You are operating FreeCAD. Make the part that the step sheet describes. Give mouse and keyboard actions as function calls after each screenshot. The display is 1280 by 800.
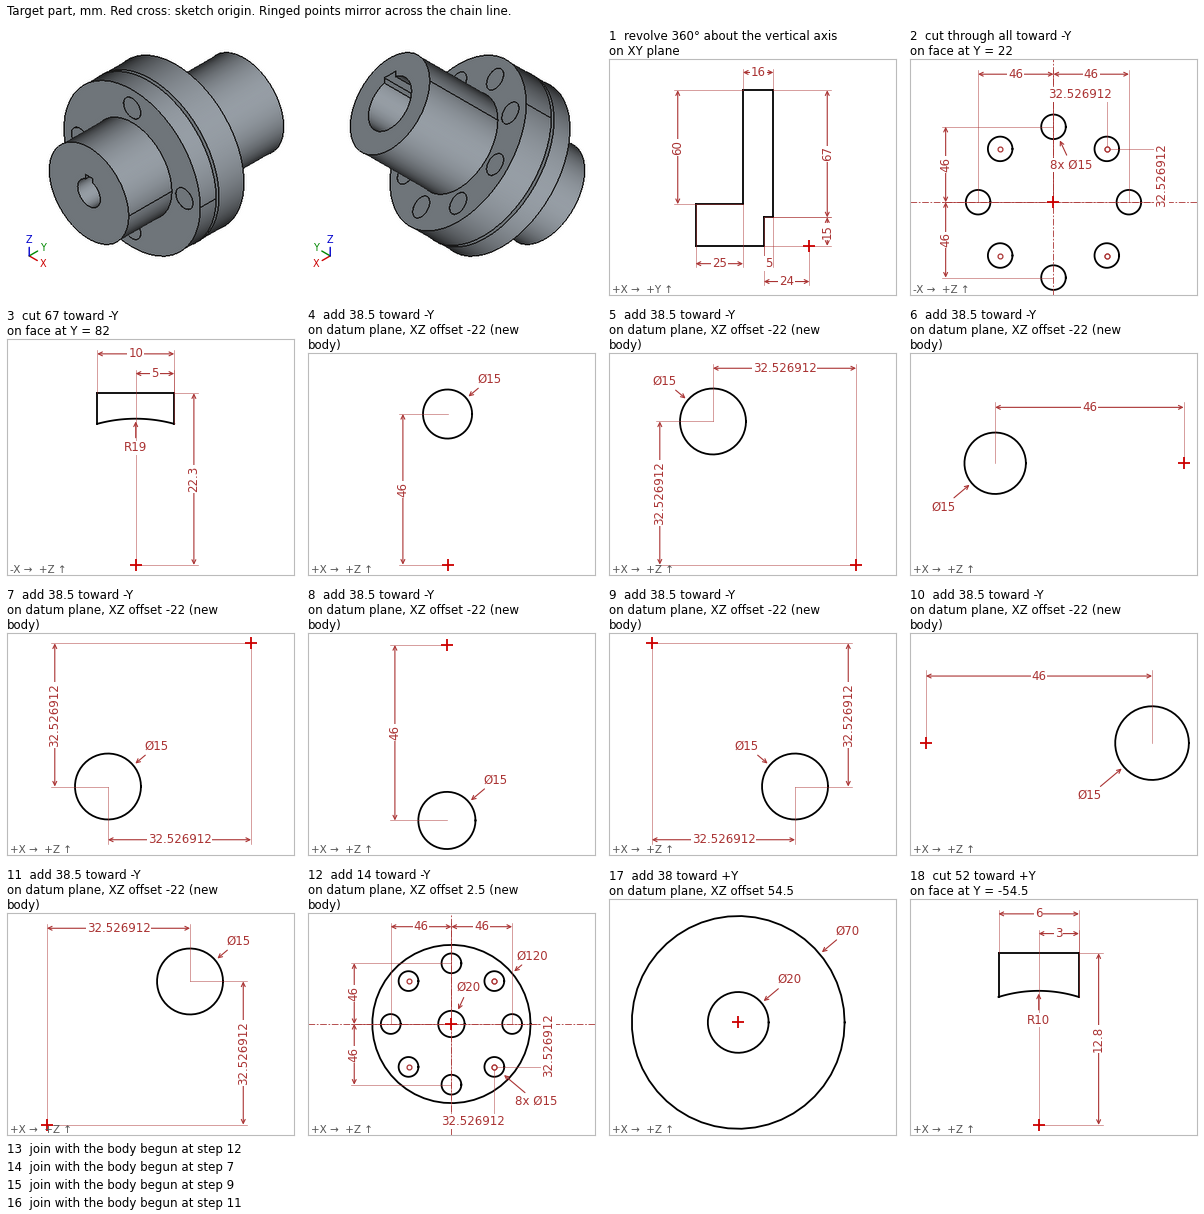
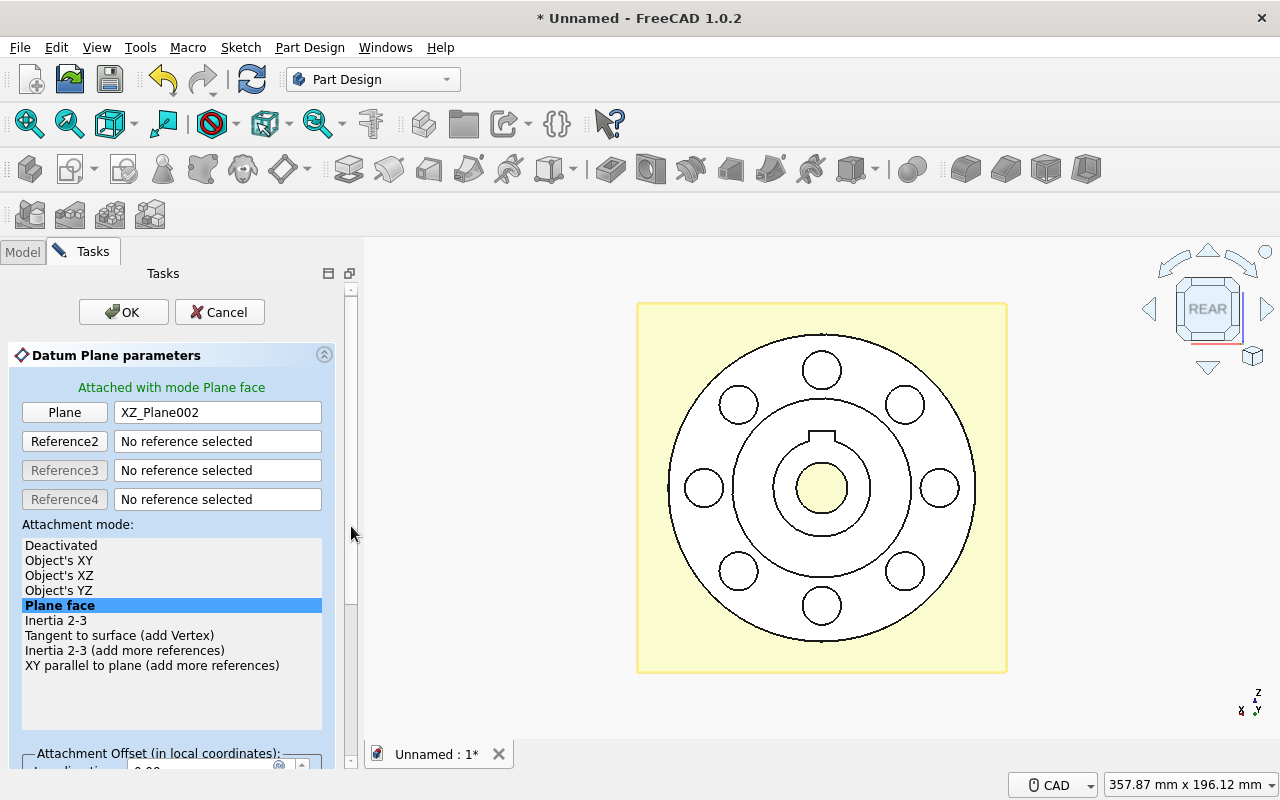
click(124, 312)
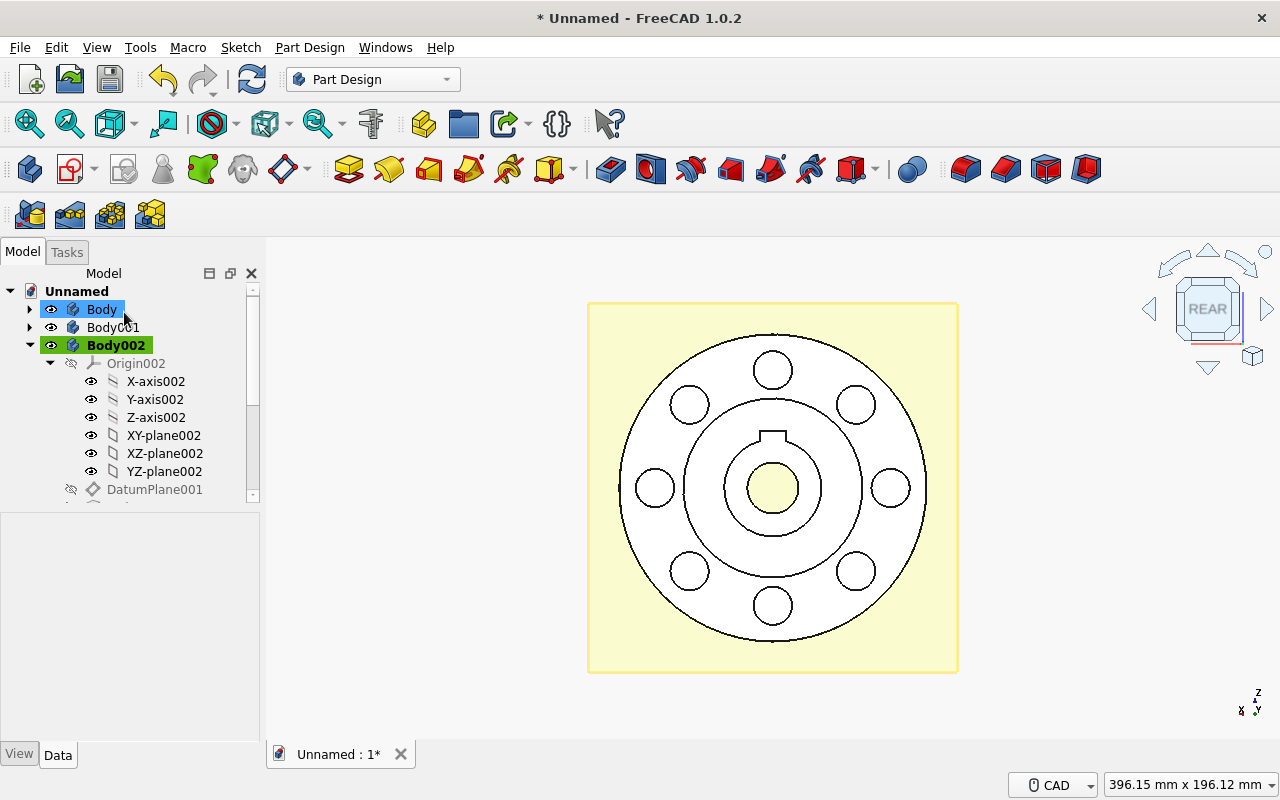
scroll(100, 395, down, 3)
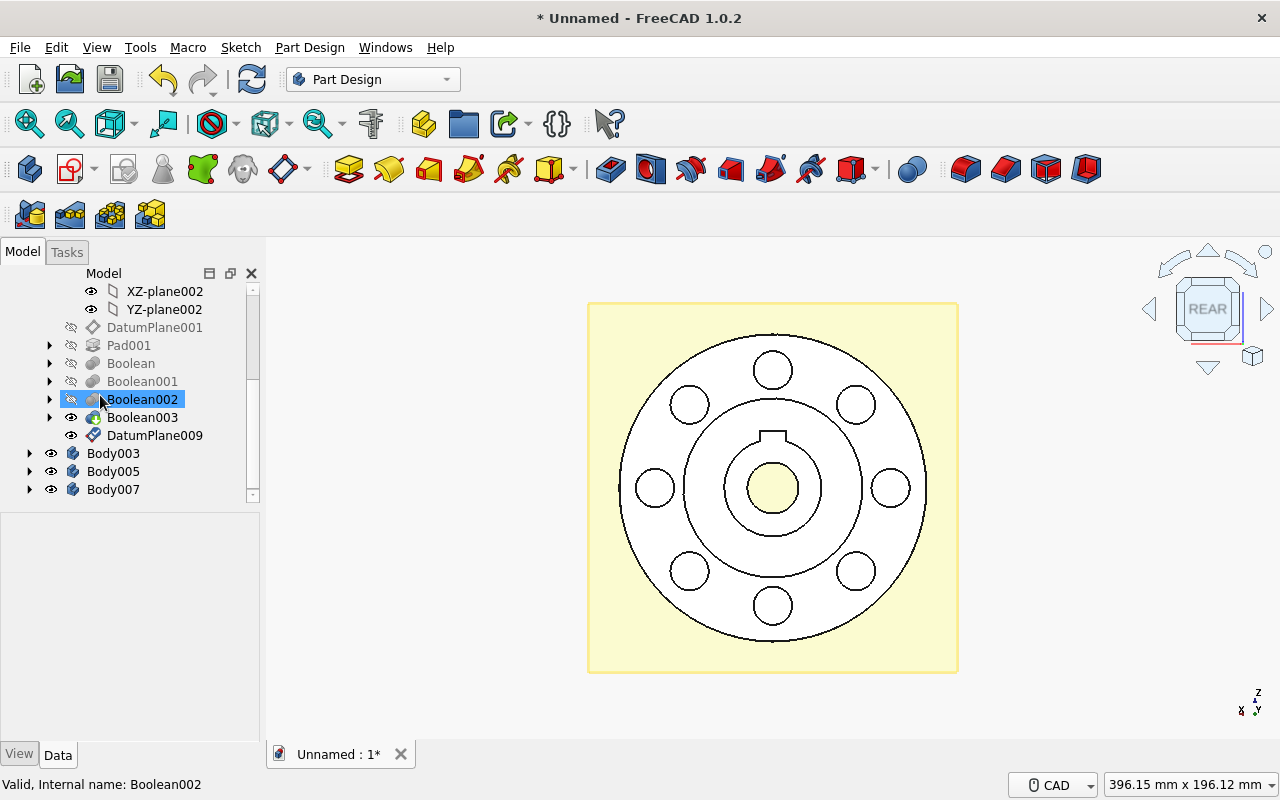
click(116, 435)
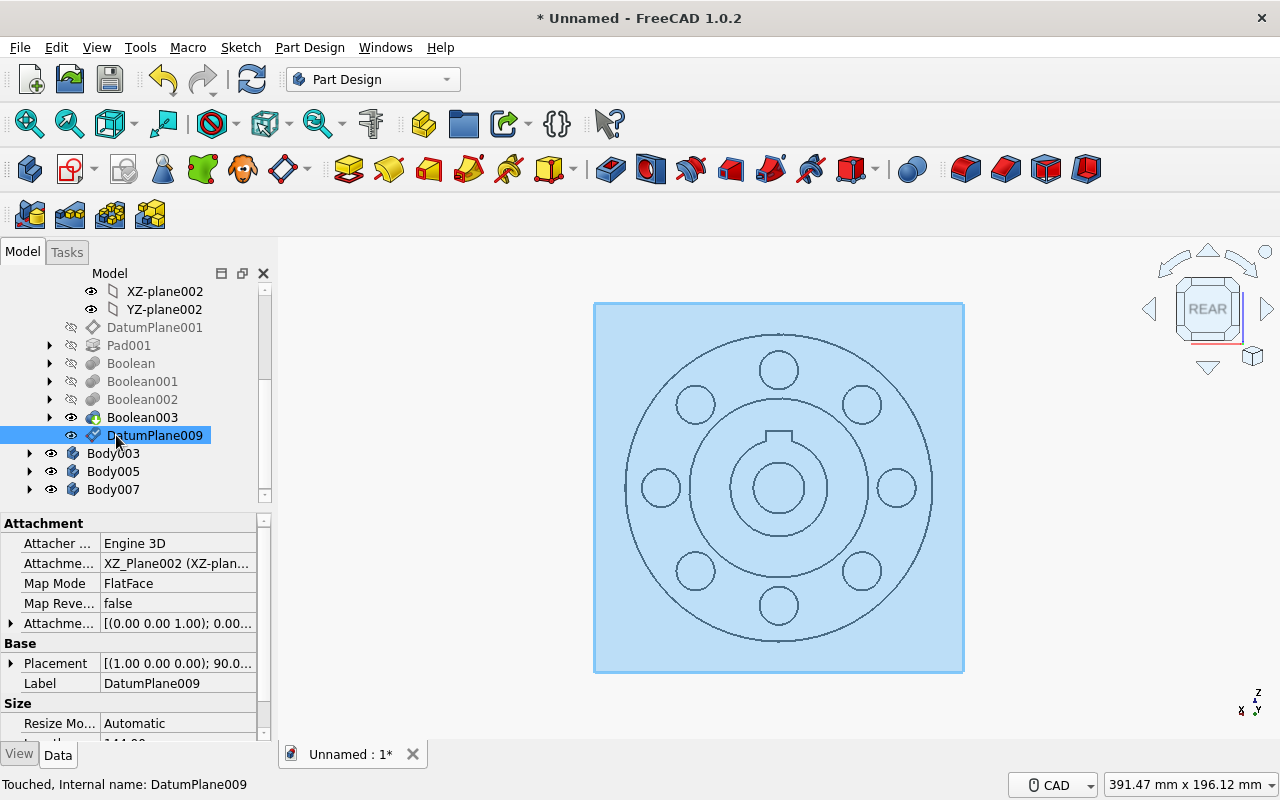
click(70, 170)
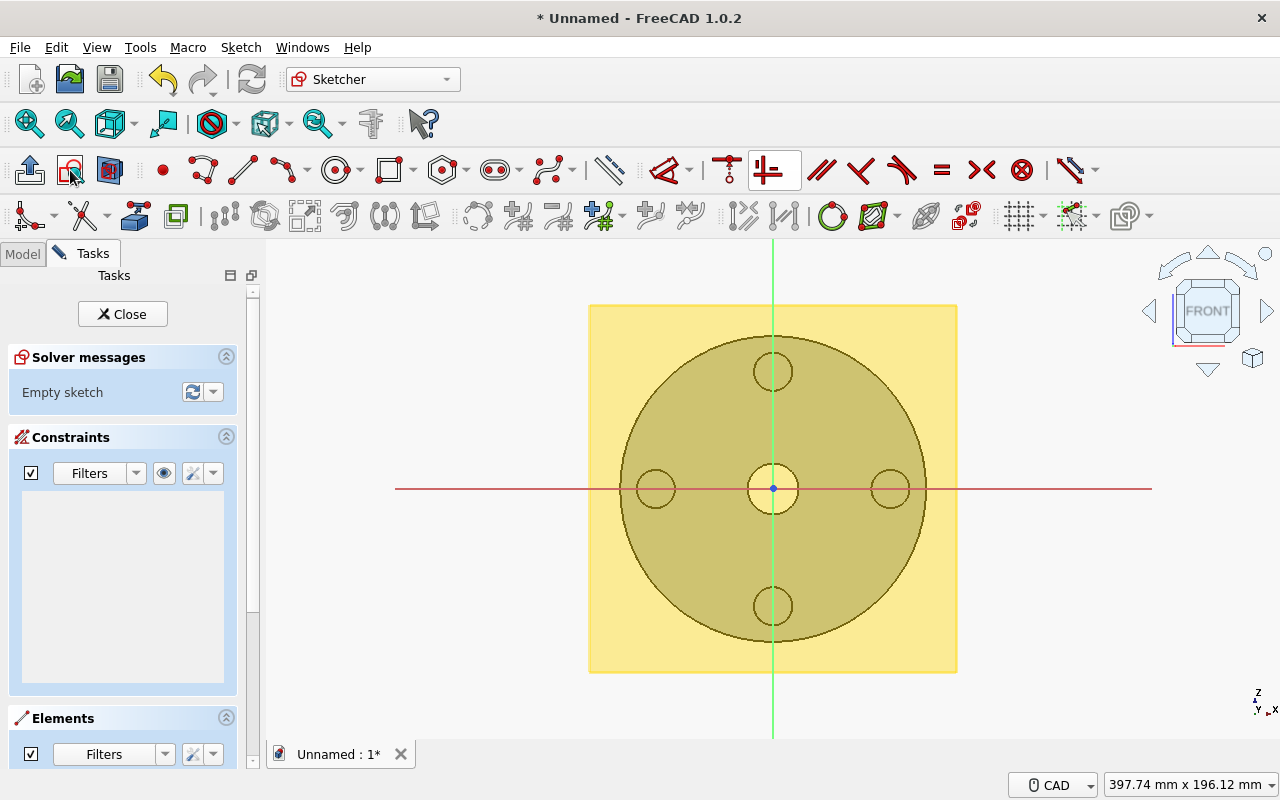
scroll(857, 489, up, 3)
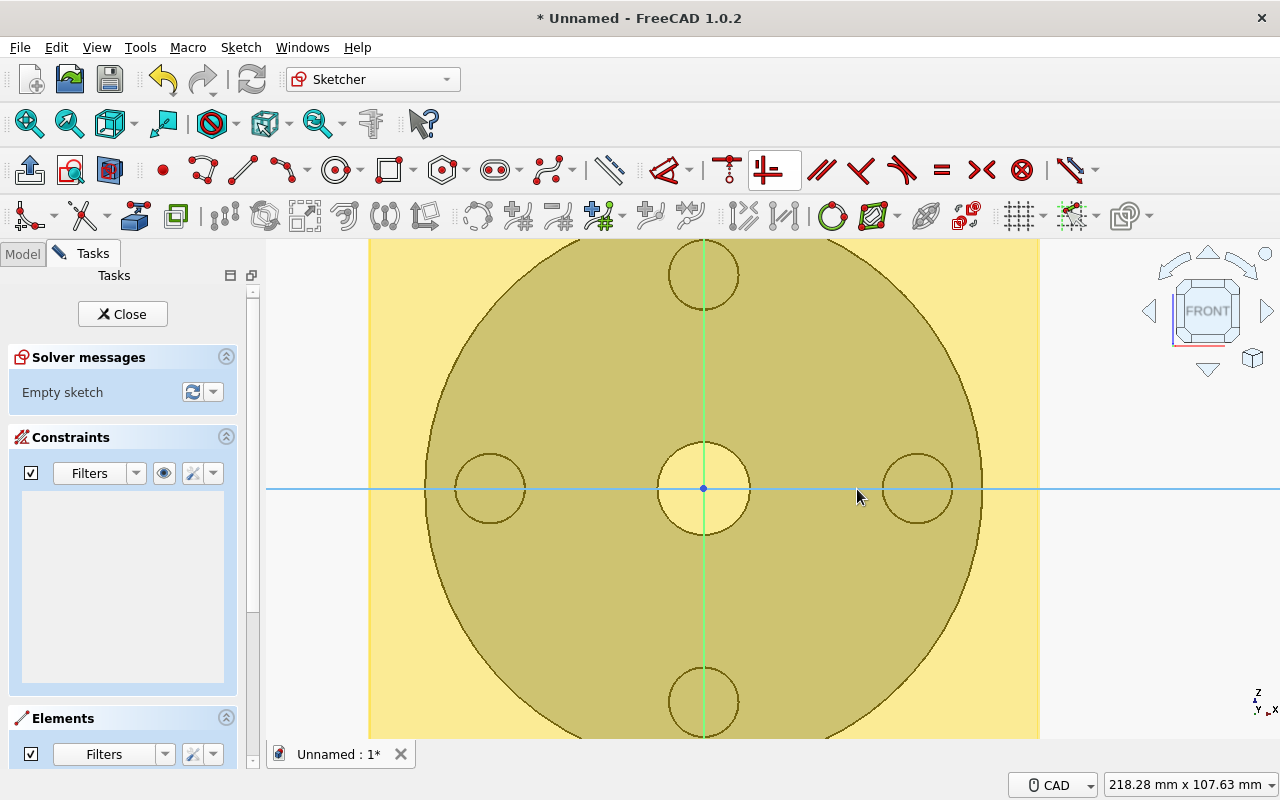
click(336, 170)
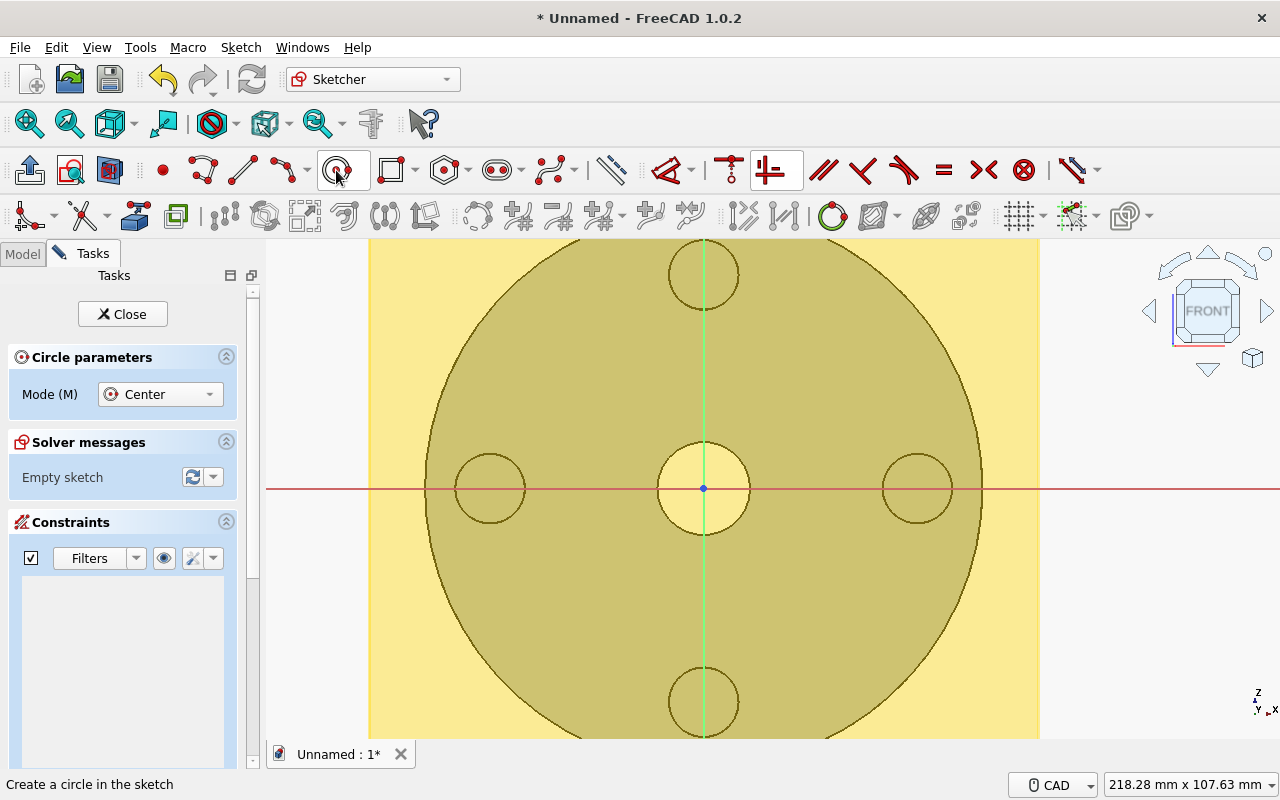
click(704, 489)
click(819, 374)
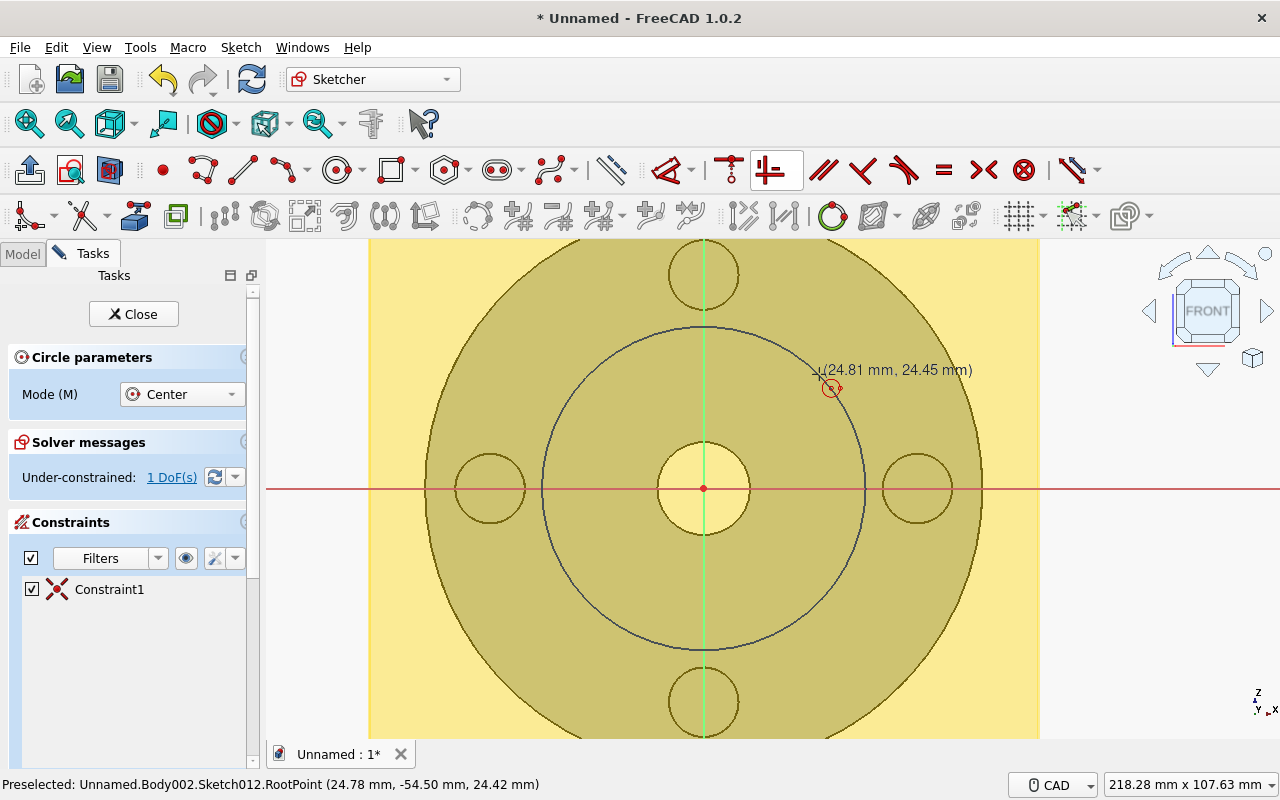
click(704, 489)
click(737, 456)
key(Escape)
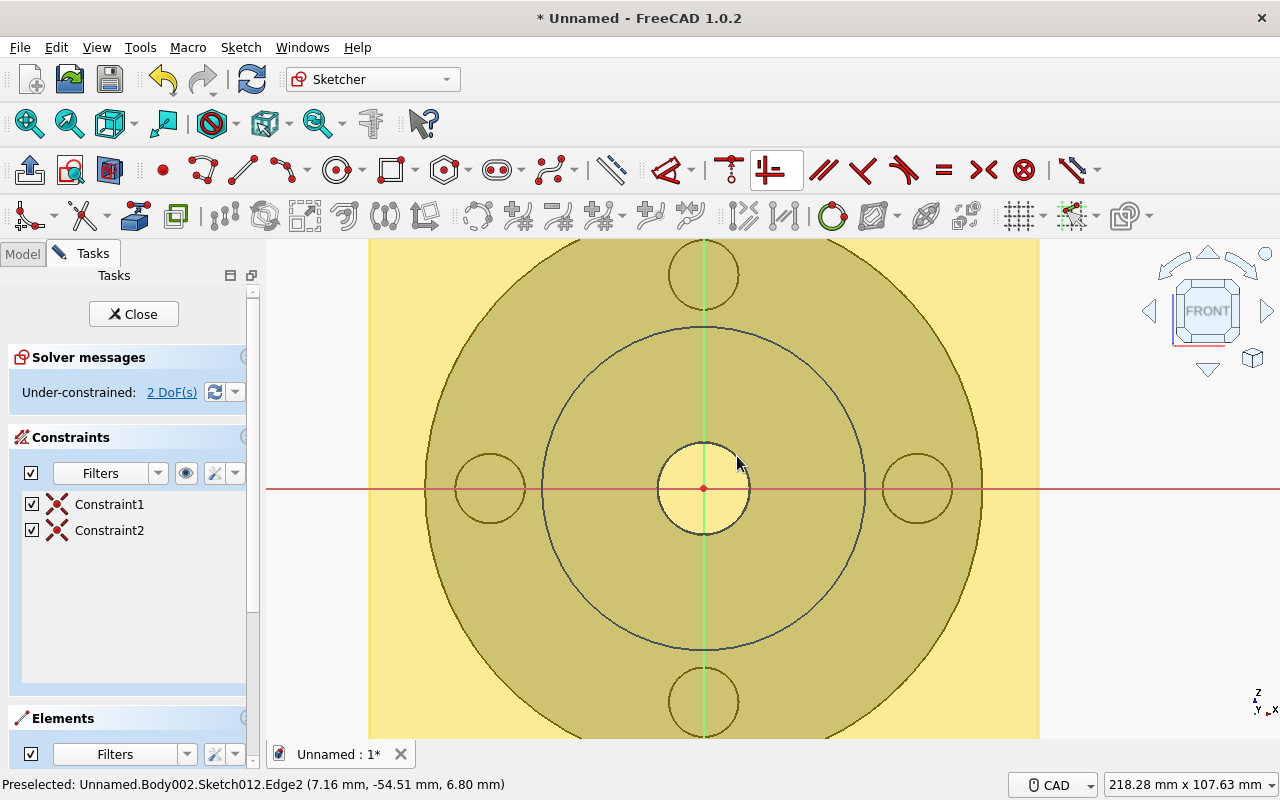
click(666, 170)